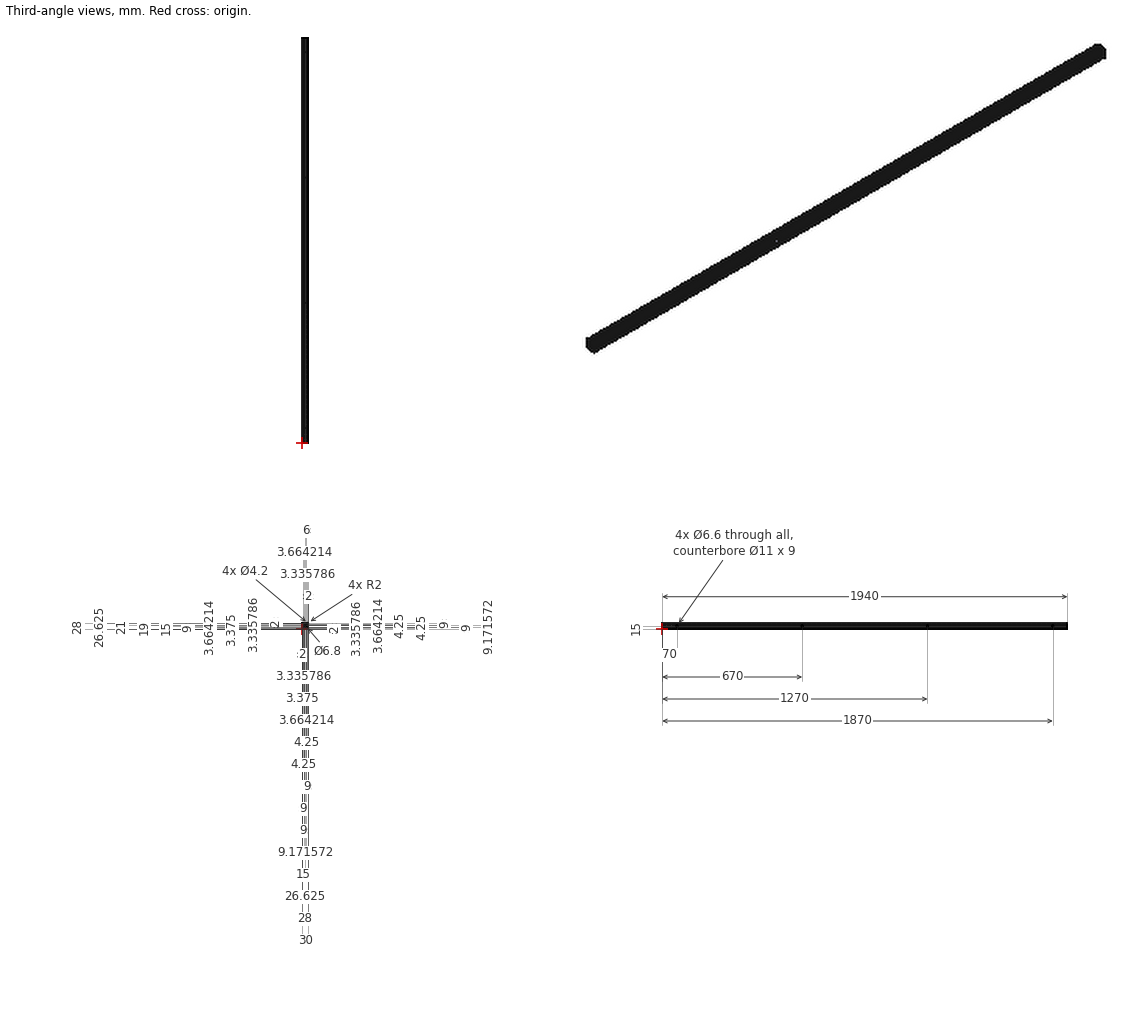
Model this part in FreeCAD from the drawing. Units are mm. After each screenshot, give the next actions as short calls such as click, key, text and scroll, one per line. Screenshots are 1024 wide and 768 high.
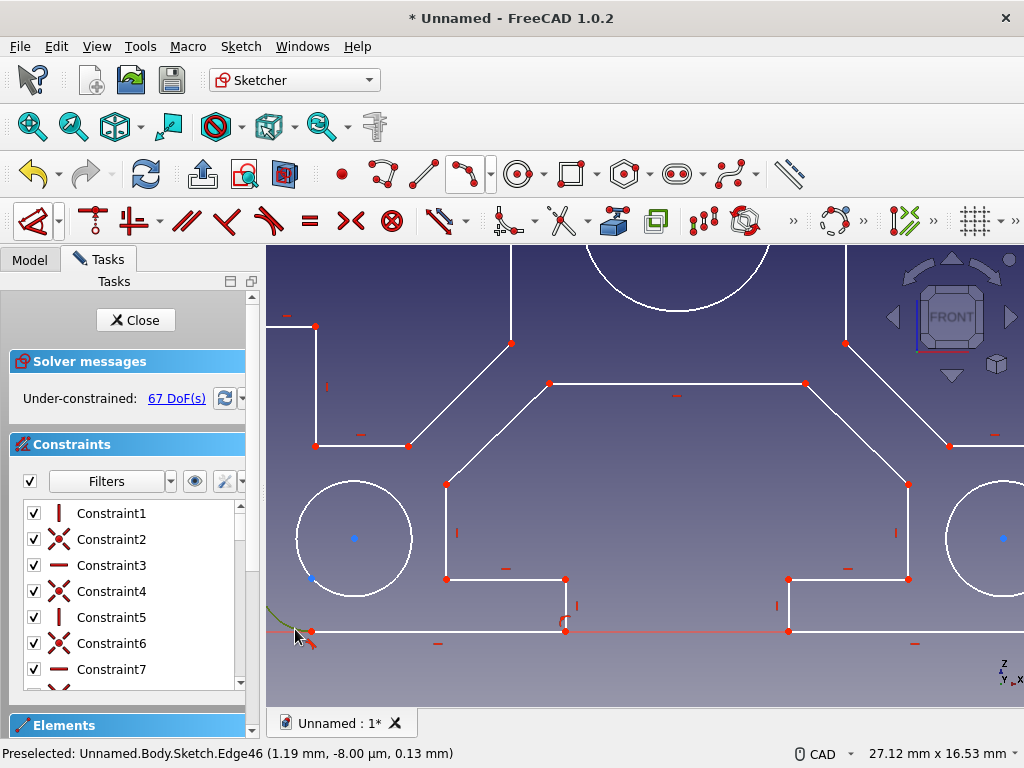
scroll(517, 629, down, 5)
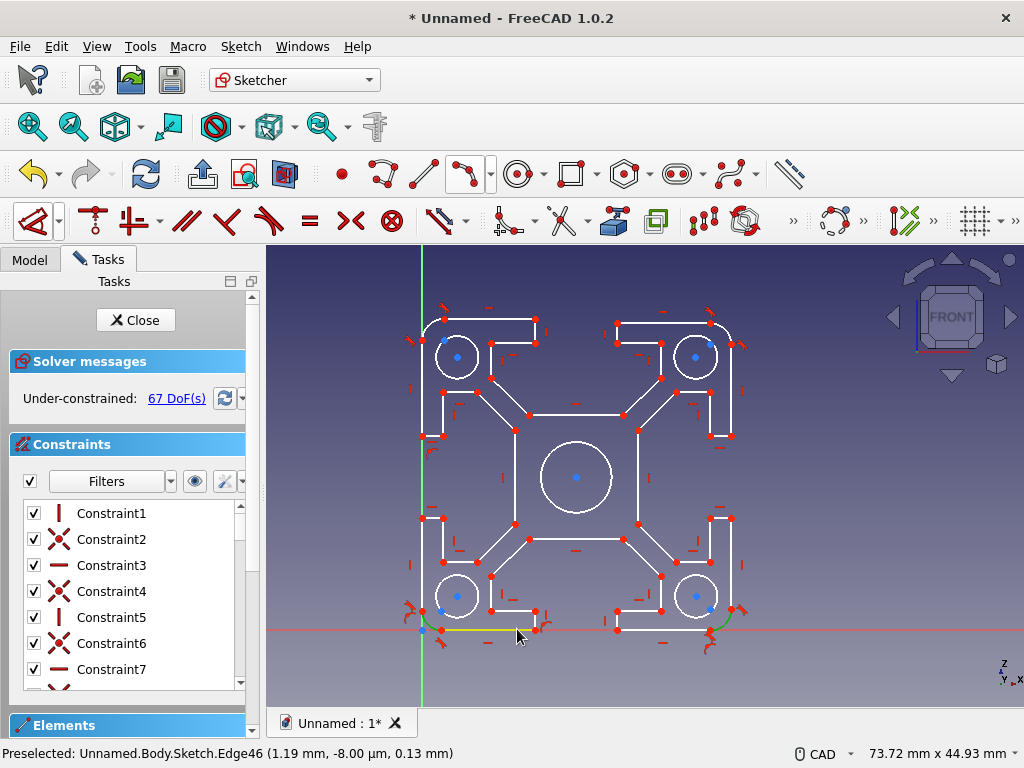
scroll(434, 321, up, 2)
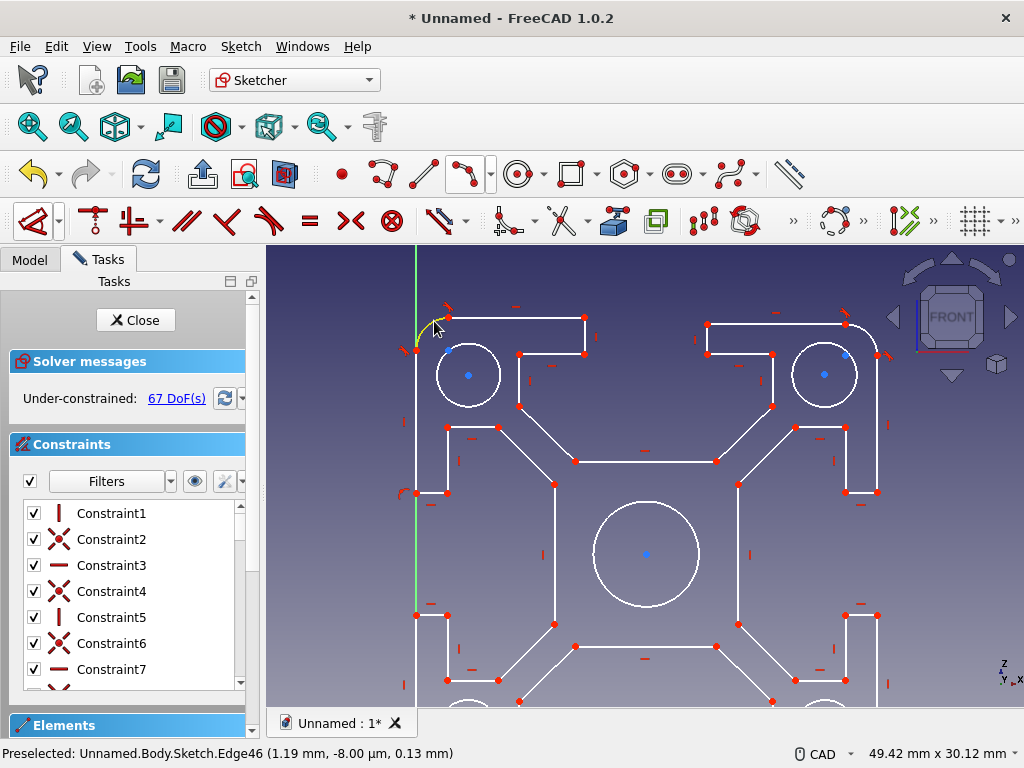
click(434, 321)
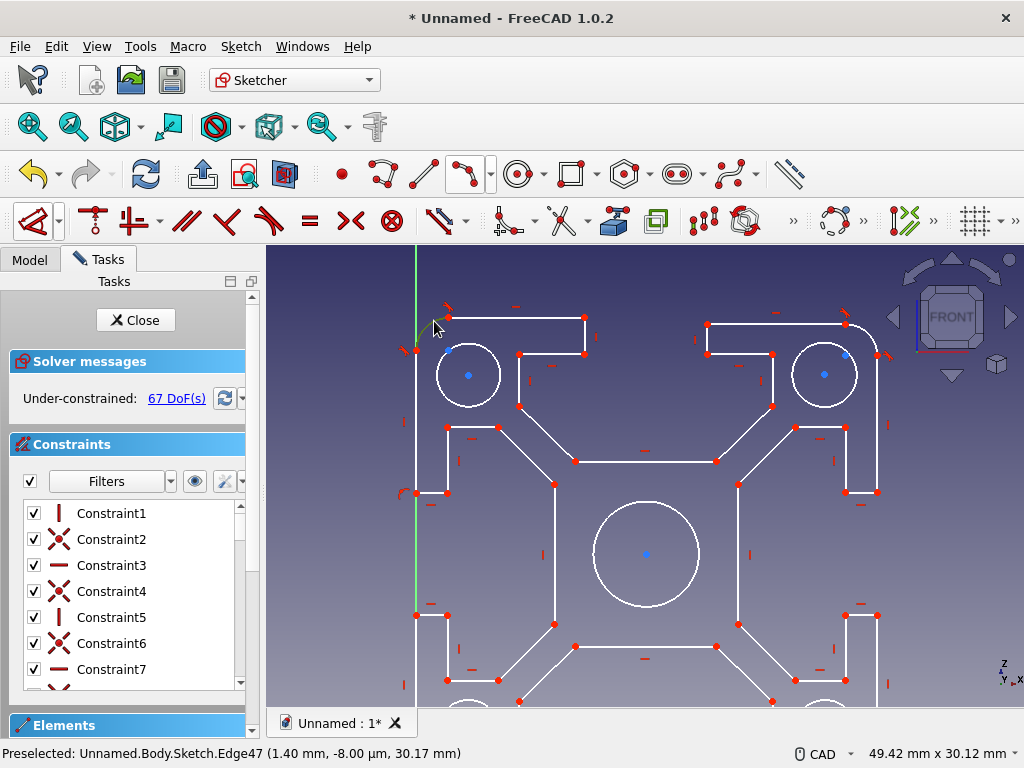
scroll(856, 326, up, 2)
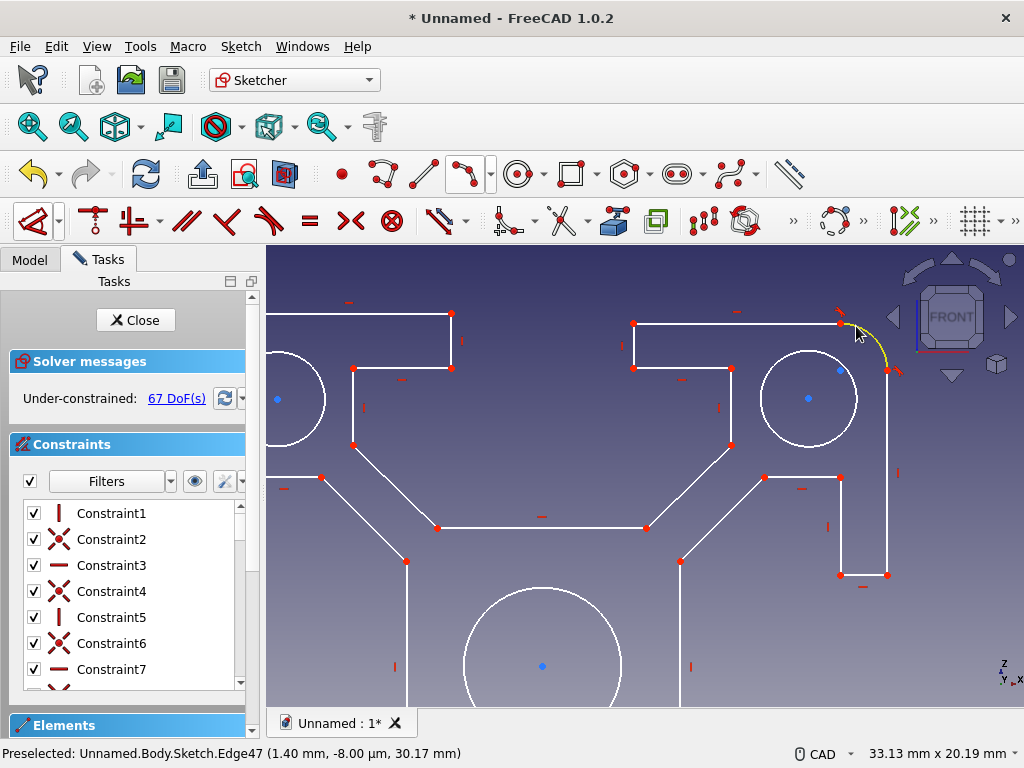
click(855, 326)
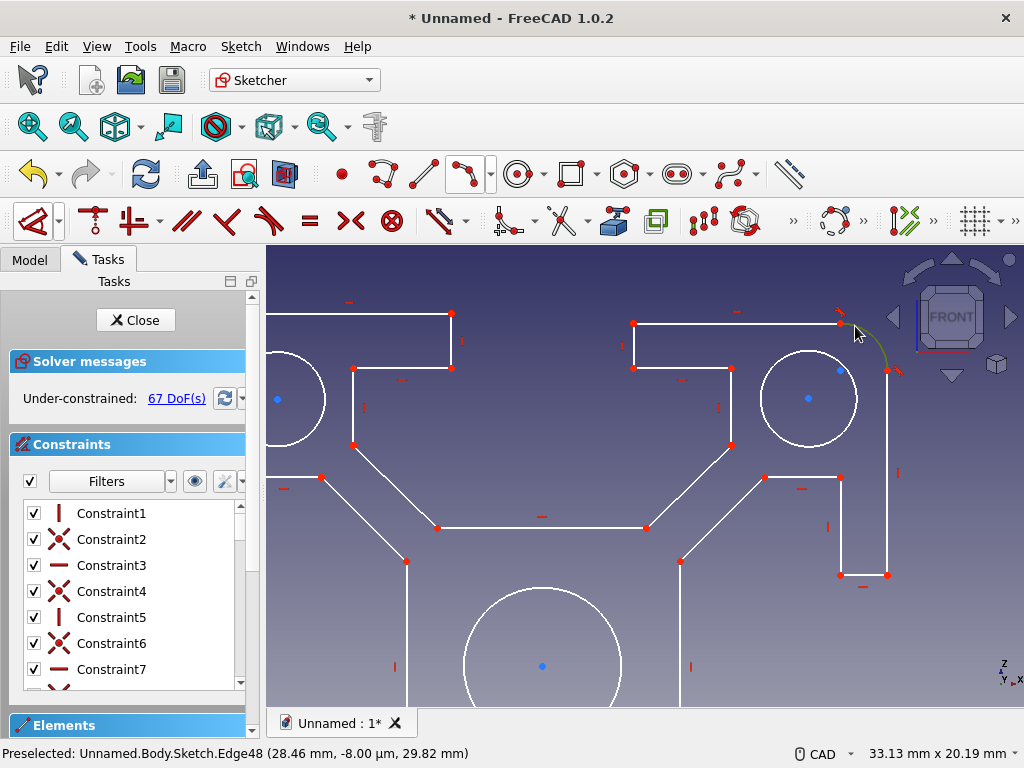
key(e)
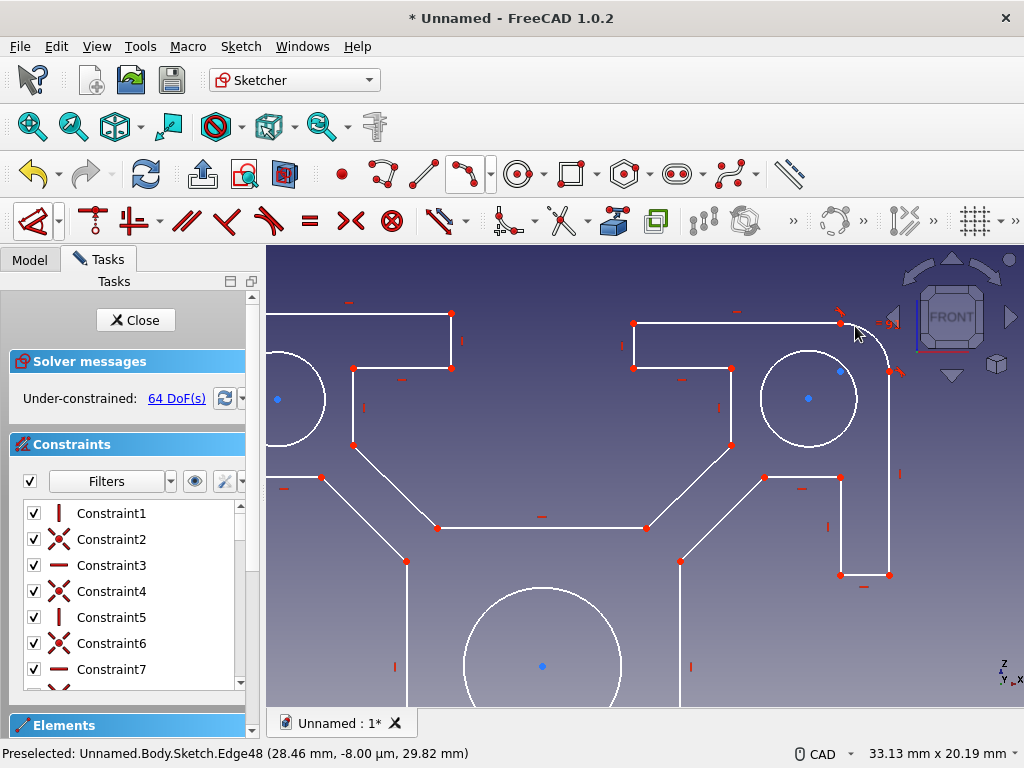
click(843, 365)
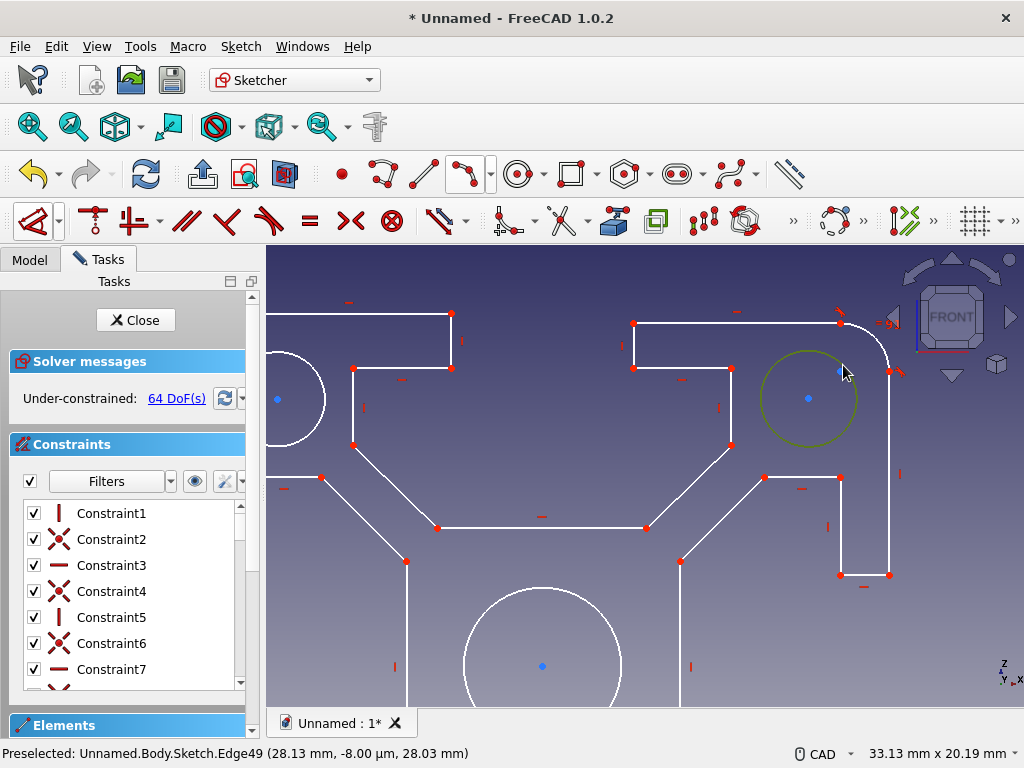
click(311, 366)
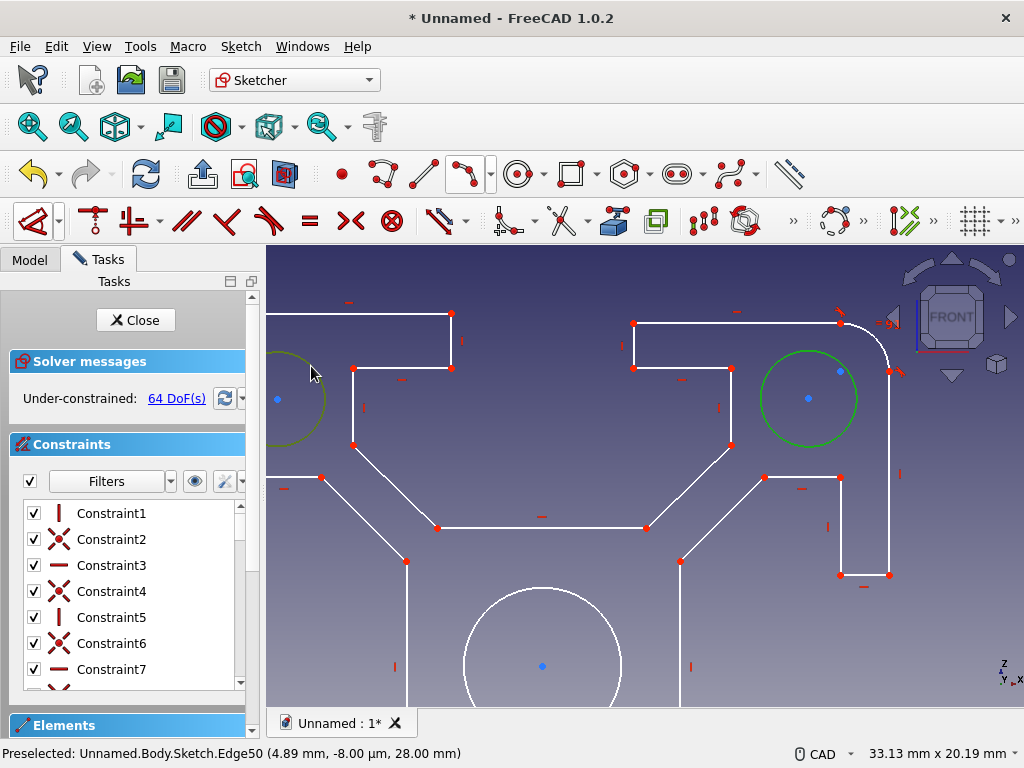
scroll(604, 323, down, 4)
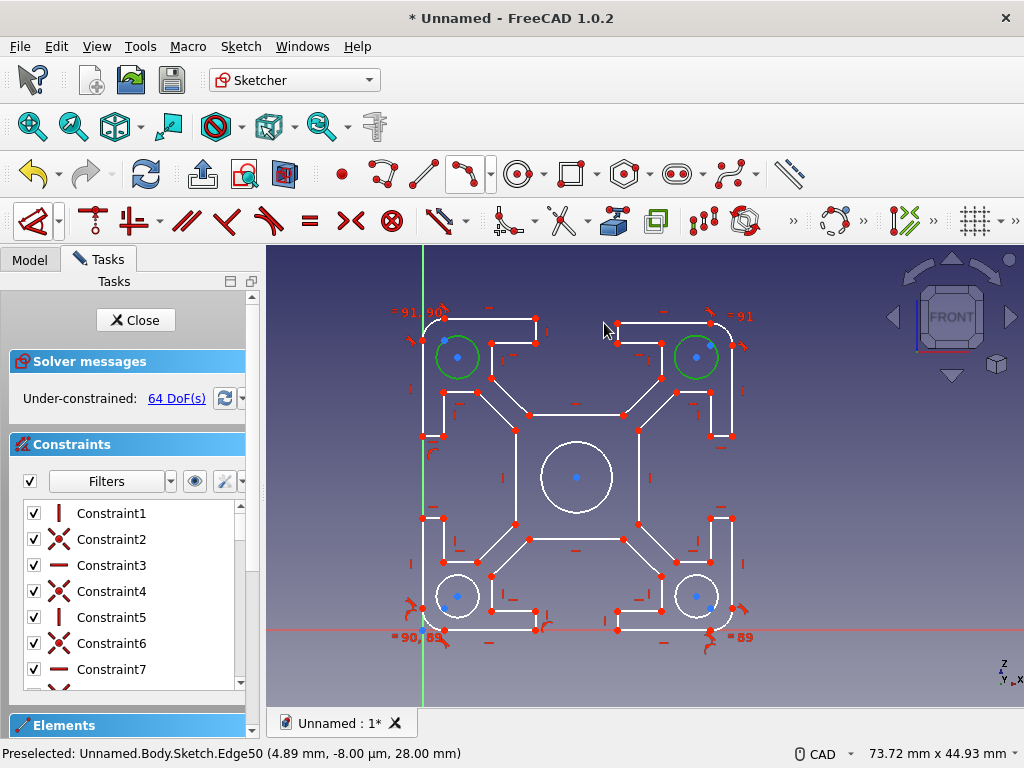
click(712, 581)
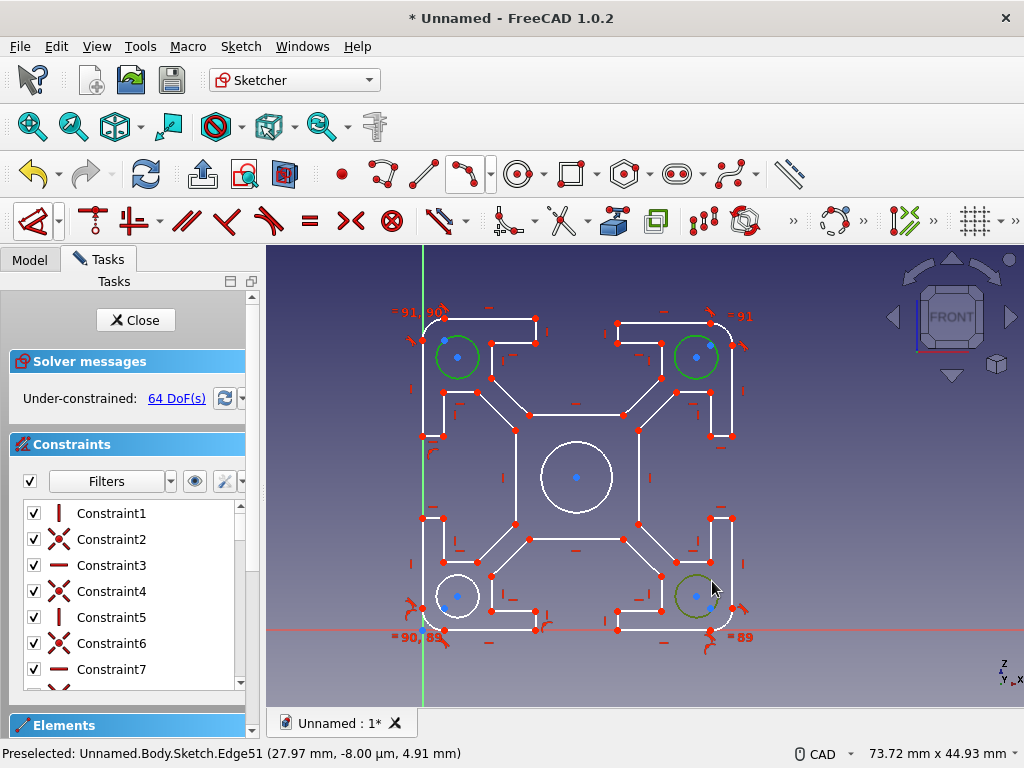
click(473, 581)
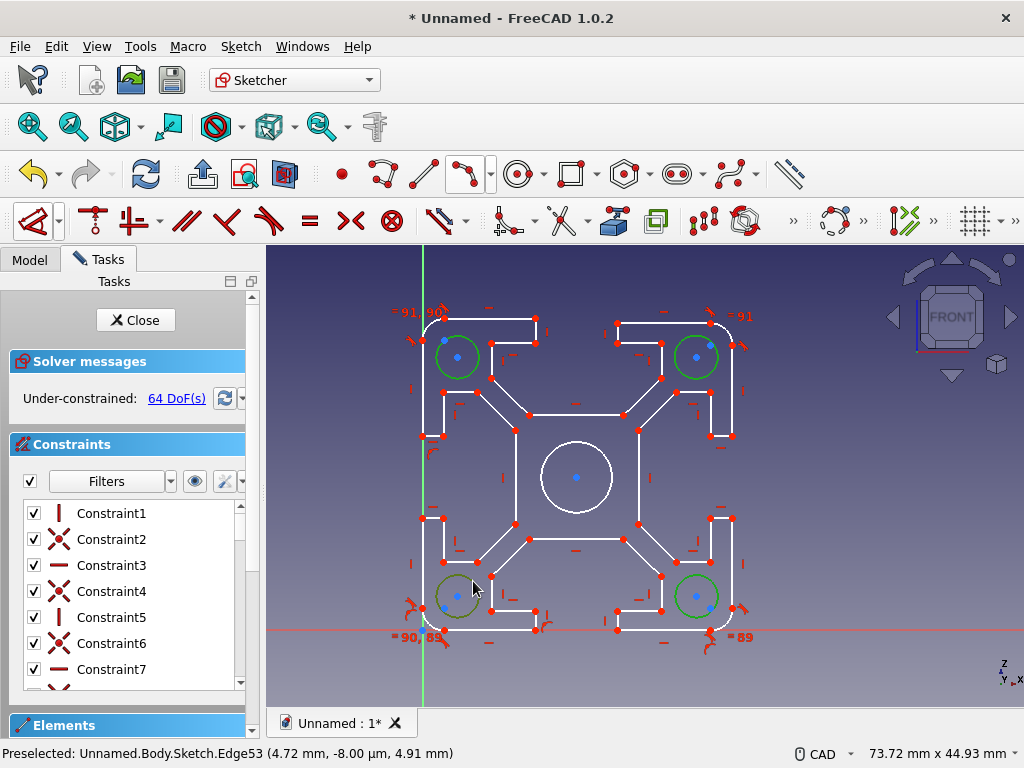
click(310, 222)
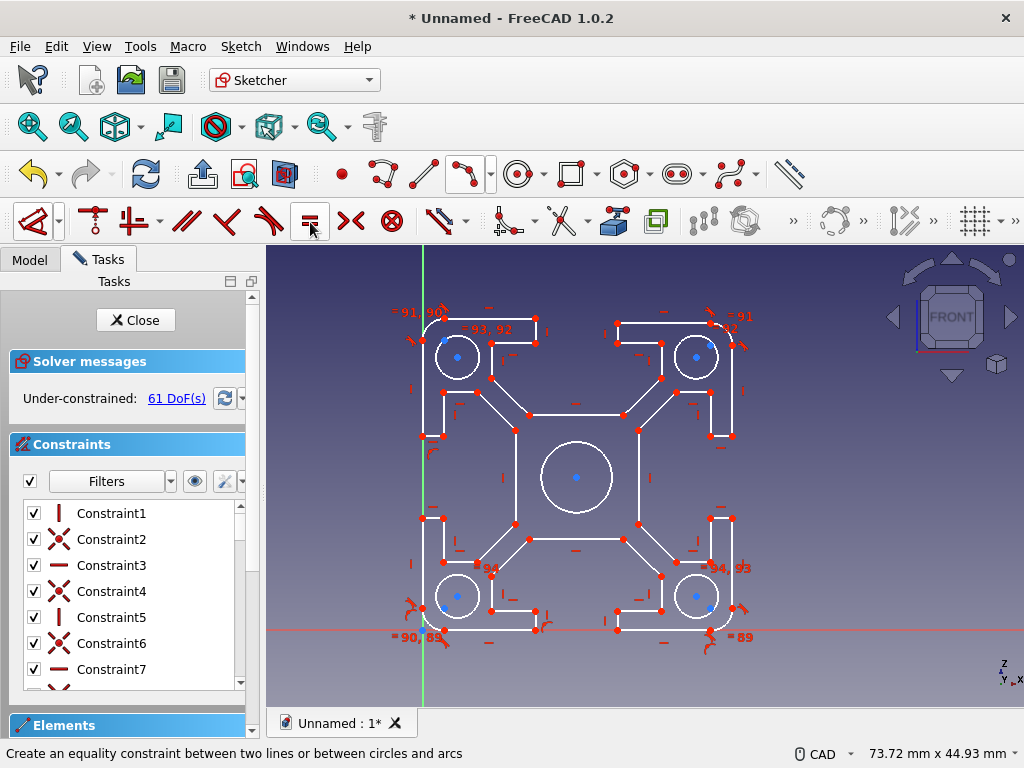
click(32, 222)